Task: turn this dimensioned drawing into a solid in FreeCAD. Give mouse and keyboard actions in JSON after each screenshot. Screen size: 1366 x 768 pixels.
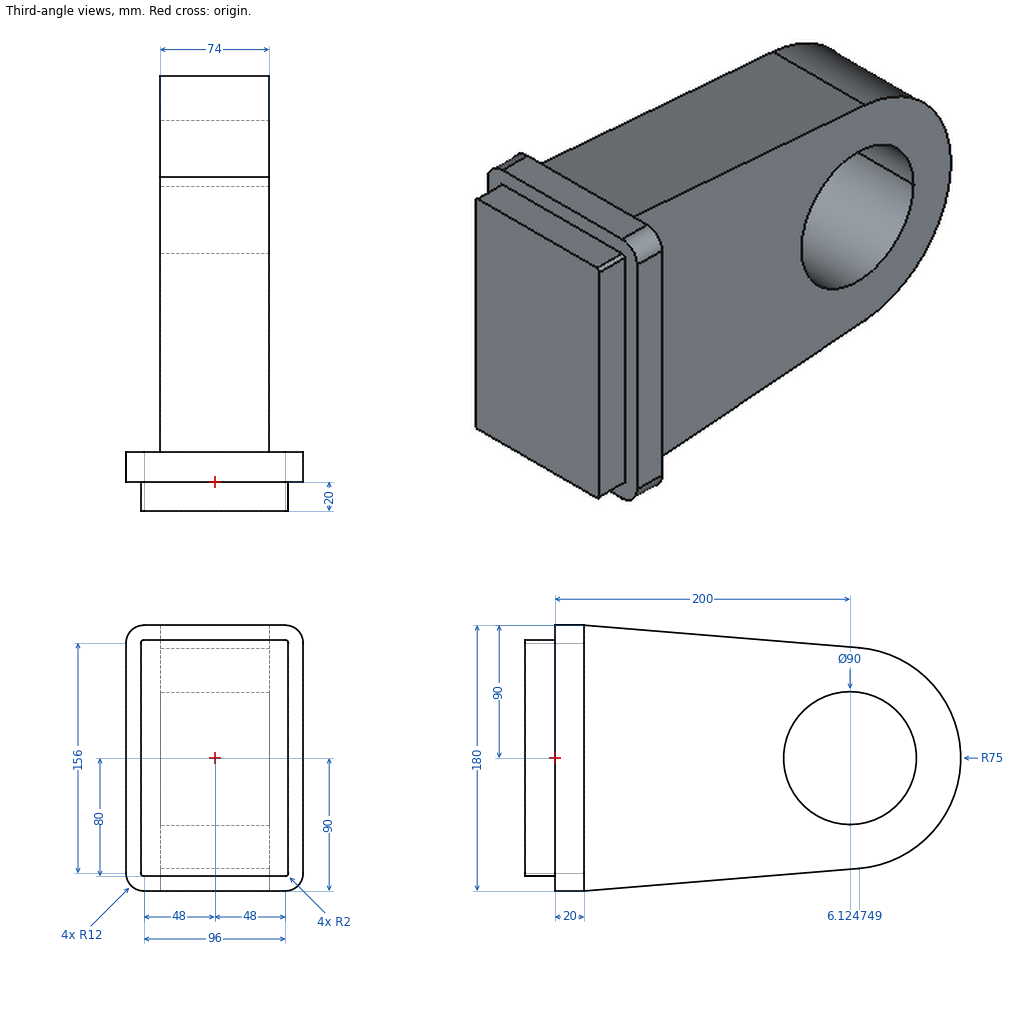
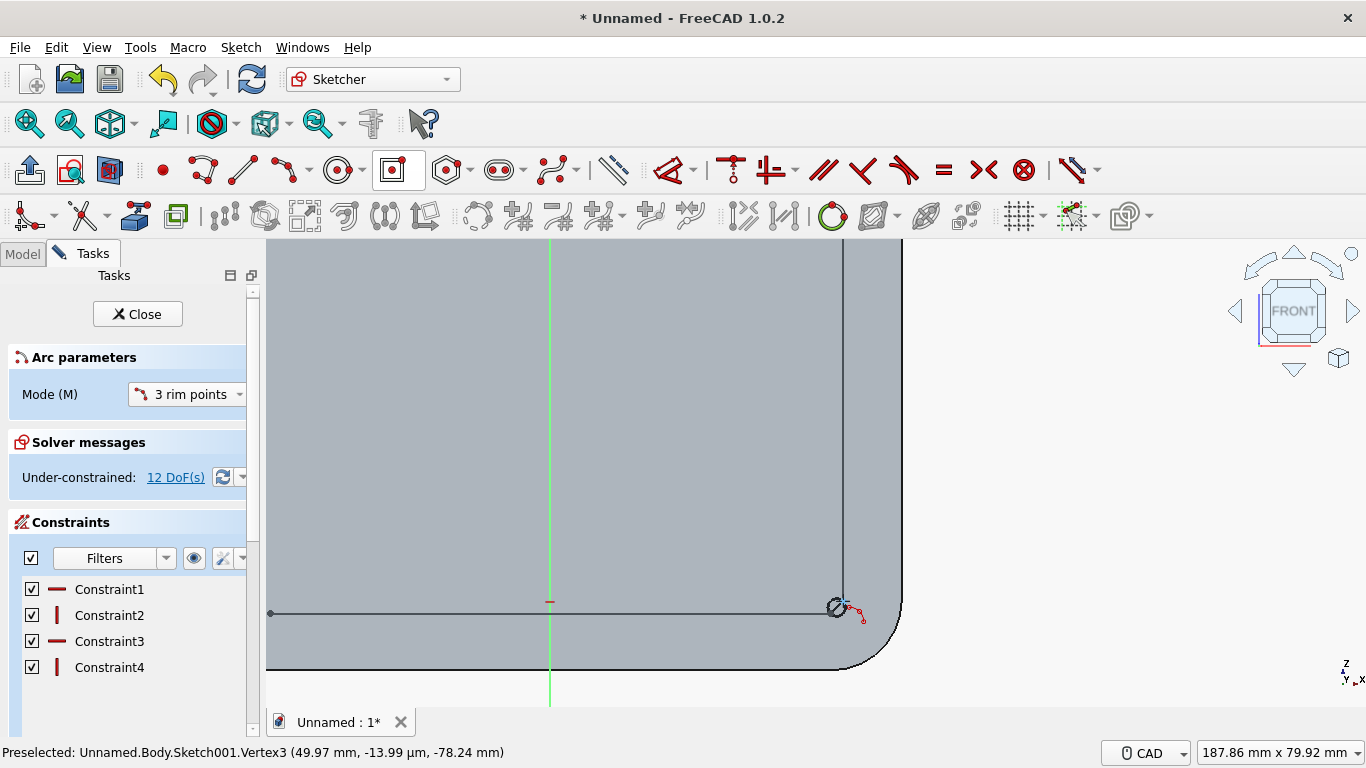
{"action": "scroll", "coordinate": [840, 608], "scroll_direction": "up", "scroll_amount": 8}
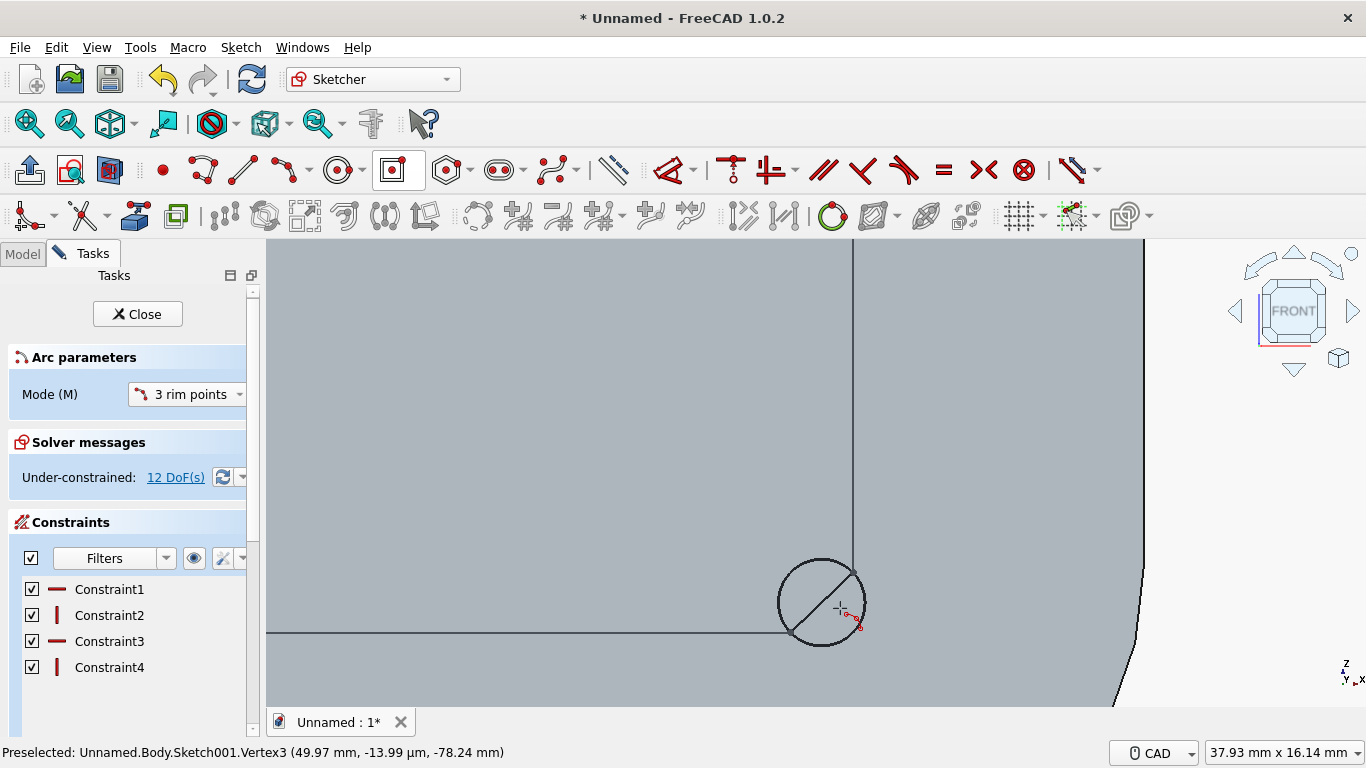
{"action": "left_click", "coordinate": [837, 607]}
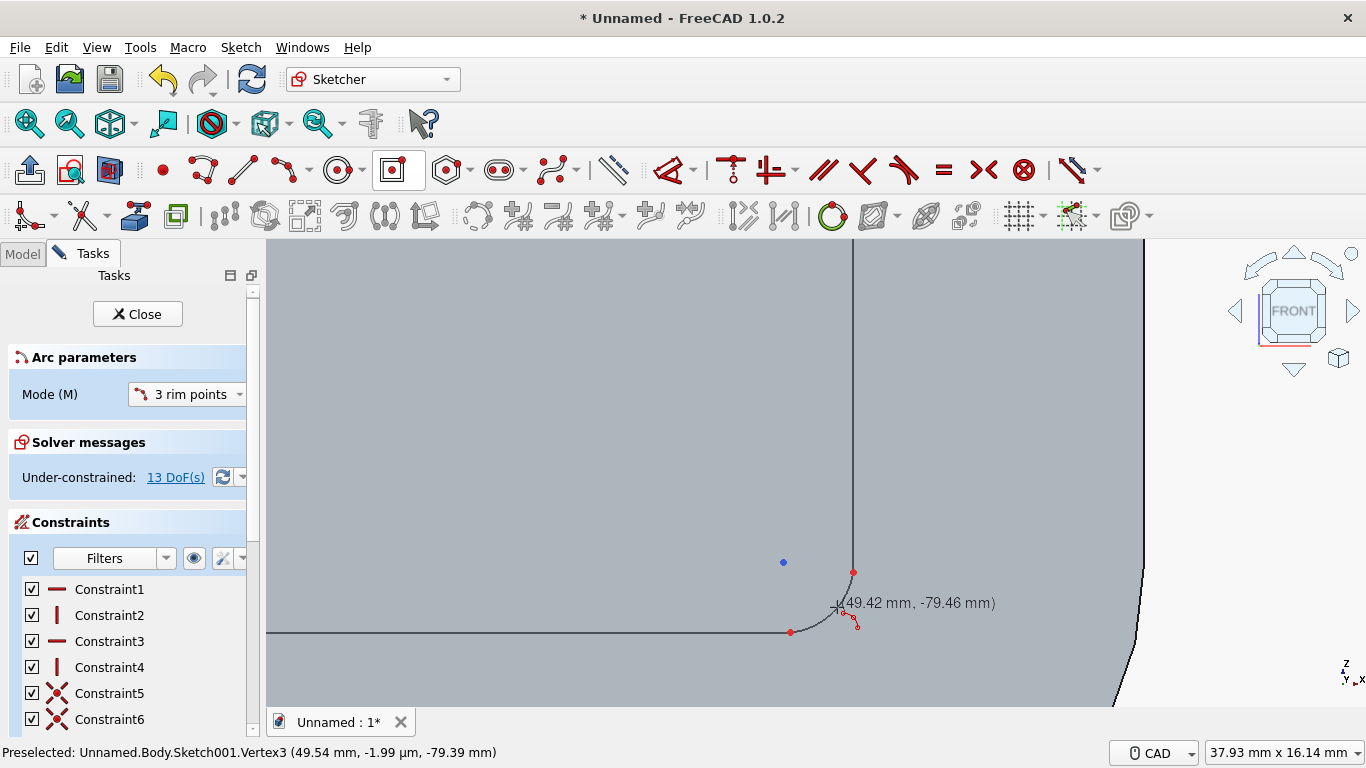
{"action": "scroll", "coordinate": [835, 613], "scroll_direction": "down", "scroll_amount": 14}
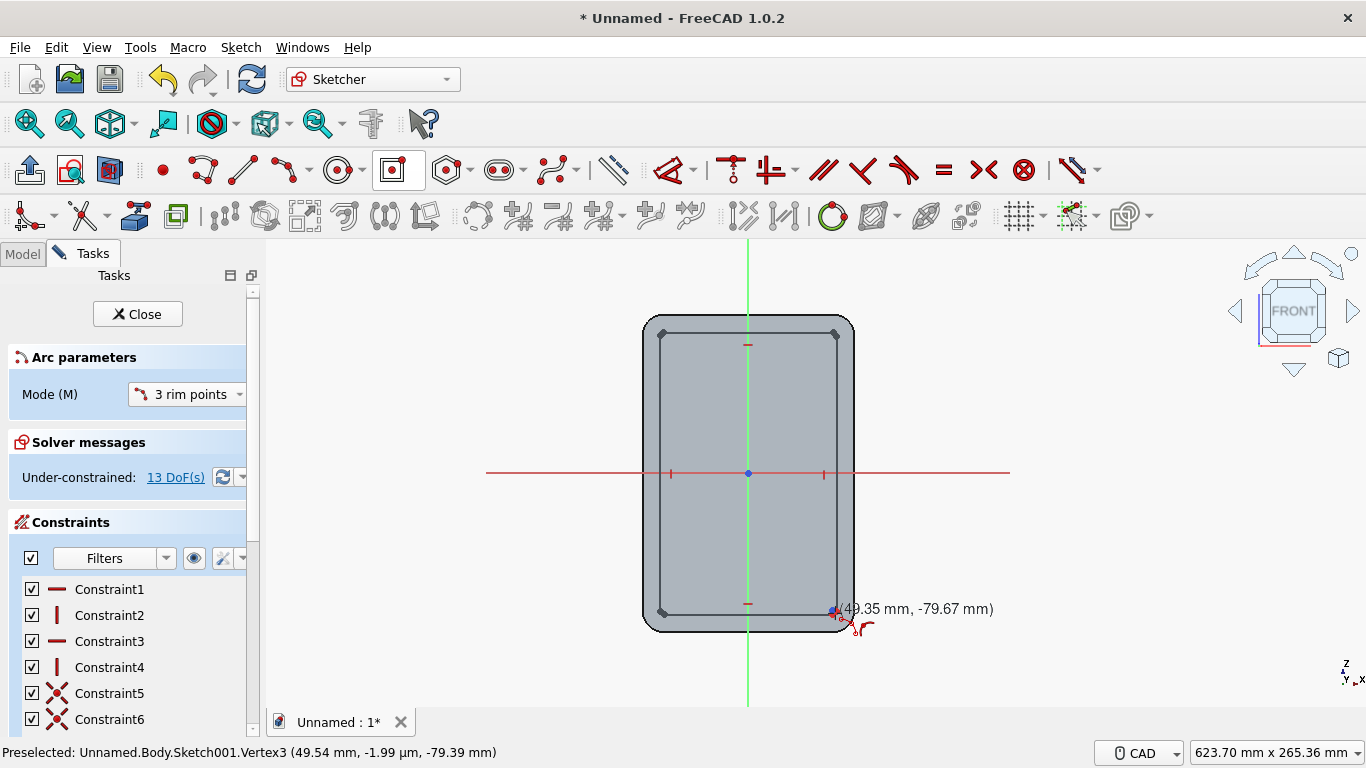
{"action": "scroll", "coordinate": [837, 336], "scroll_direction": "up", "scroll_amount": 6}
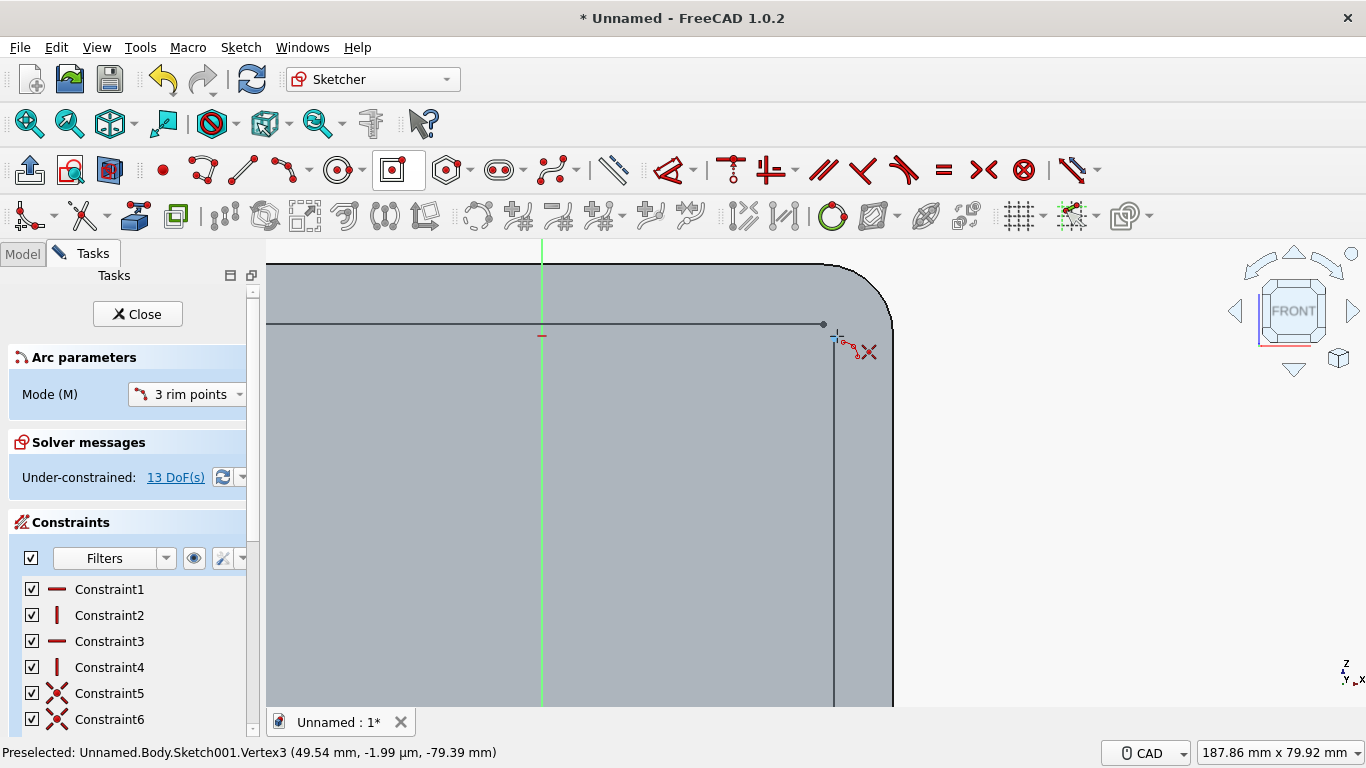
{"action": "left_click", "coordinate": [834, 338]}
{"action": "left_click", "coordinate": [823, 324]}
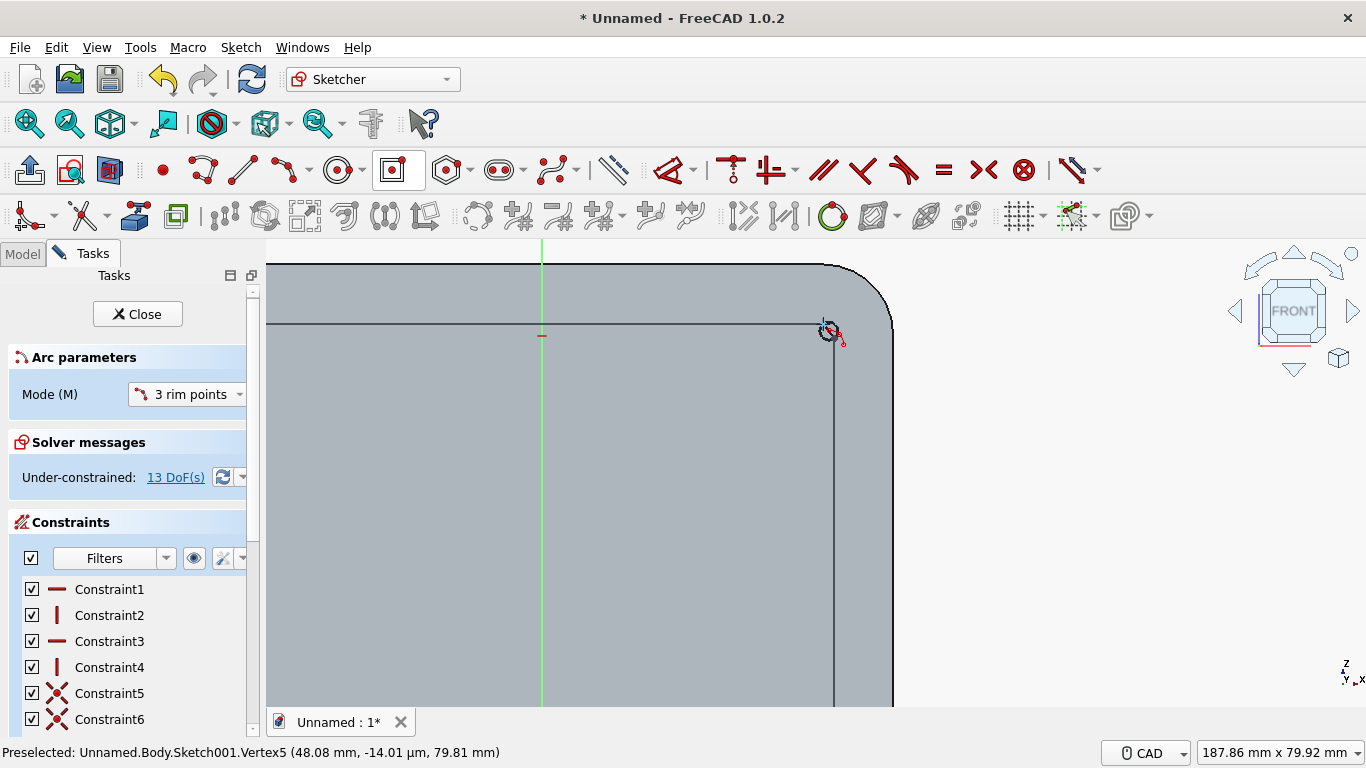
{"action": "scroll", "coordinate": [831, 326], "scroll_direction": "up", "scroll_amount": 8}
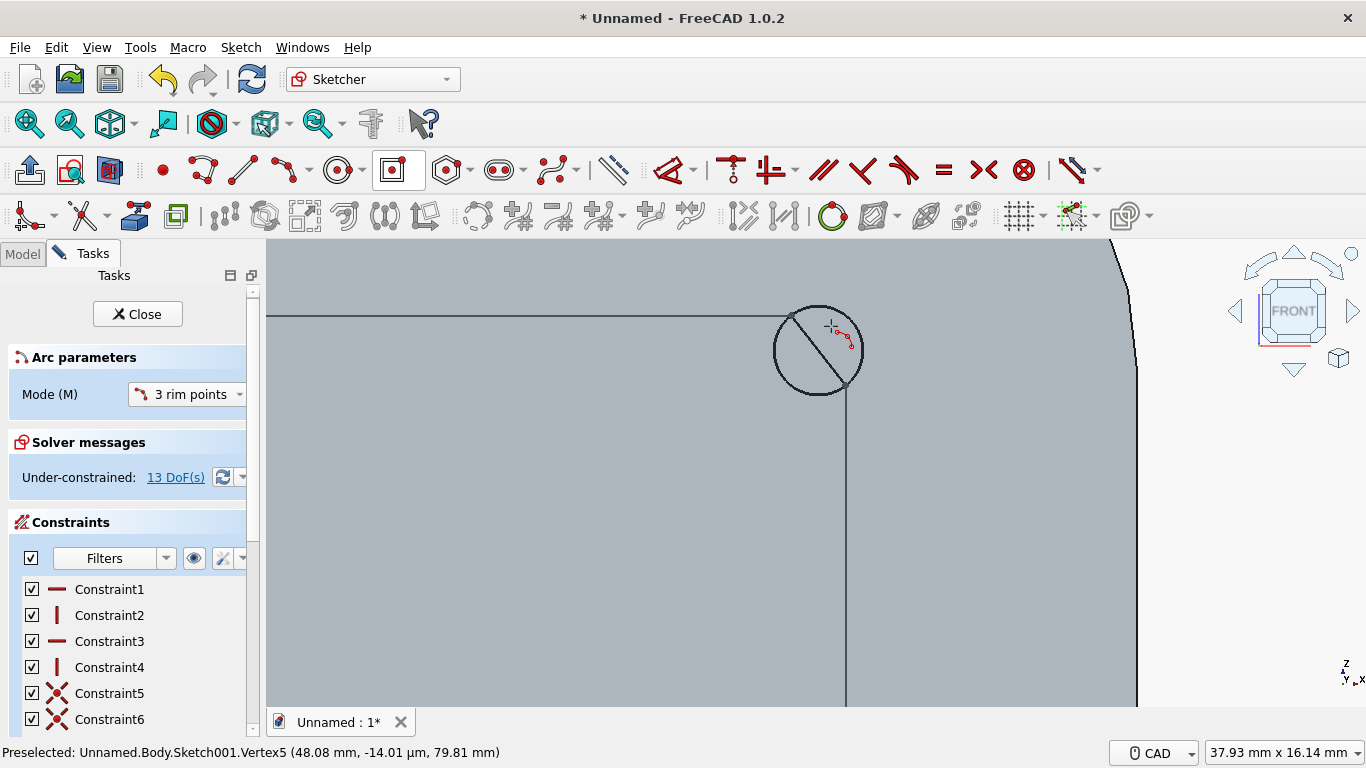
{"action": "left_click", "coordinate": [830, 327]}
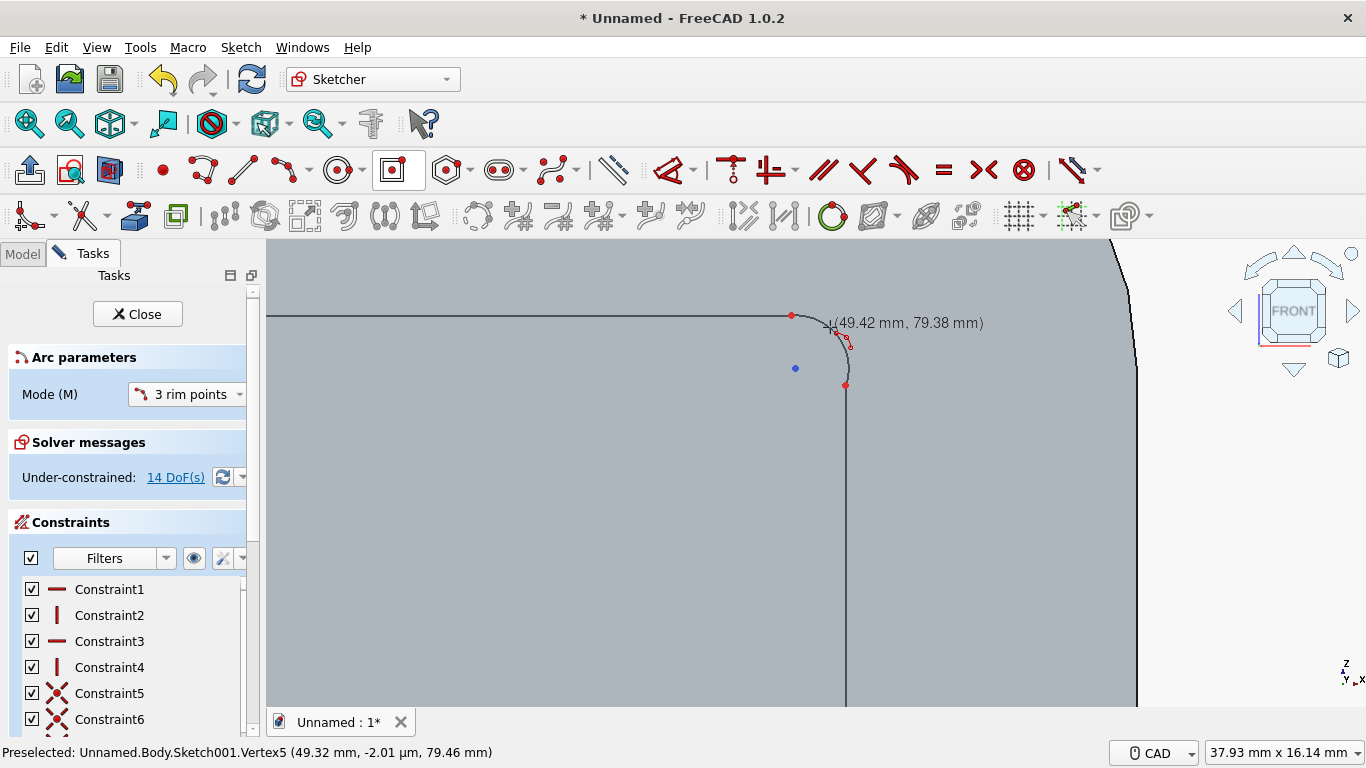
{"action": "scroll", "coordinate": [835, 333], "scroll_direction": "down", "scroll_amount": 14}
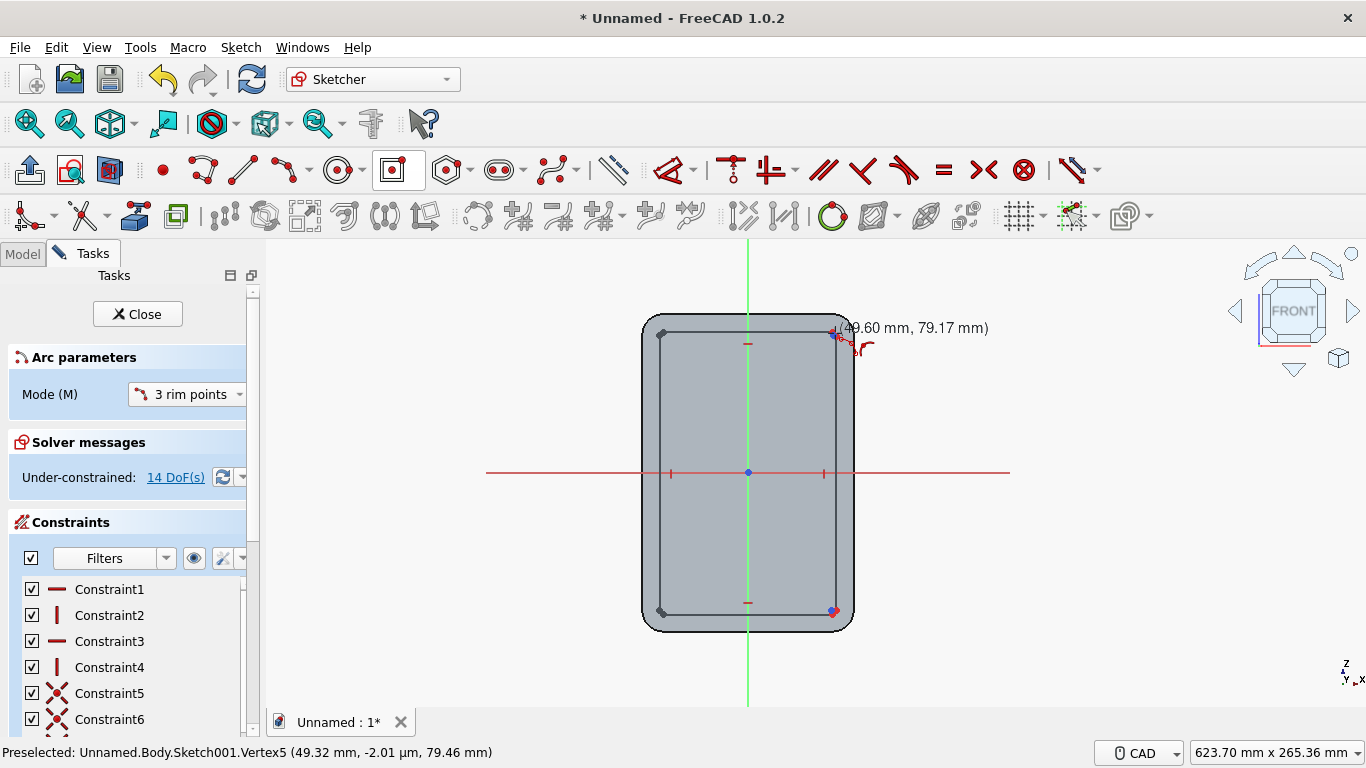
{"action": "scroll", "coordinate": [663, 332], "scroll_direction": "up", "scroll_amount": 6}